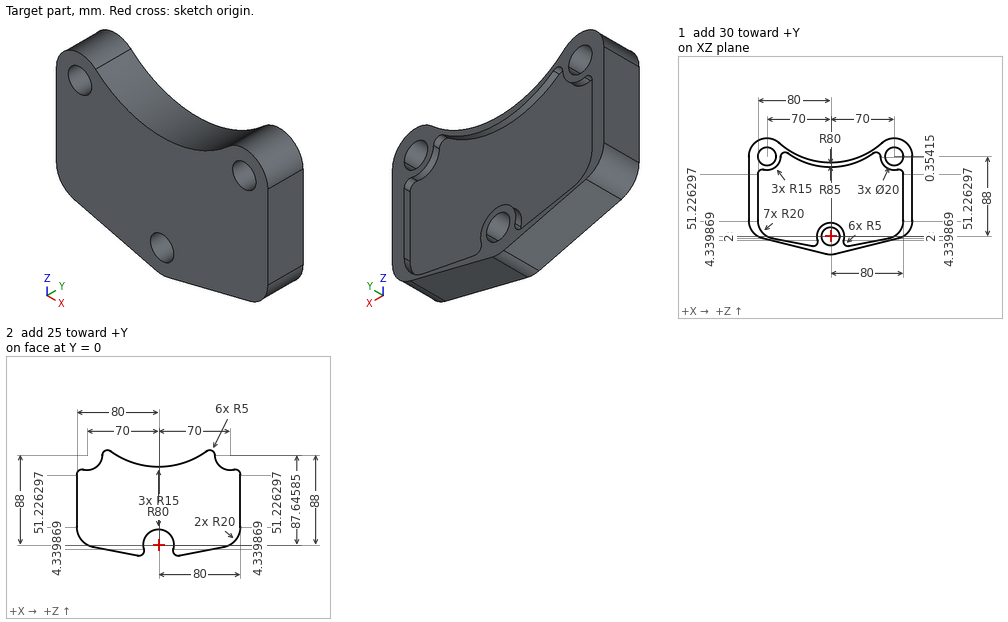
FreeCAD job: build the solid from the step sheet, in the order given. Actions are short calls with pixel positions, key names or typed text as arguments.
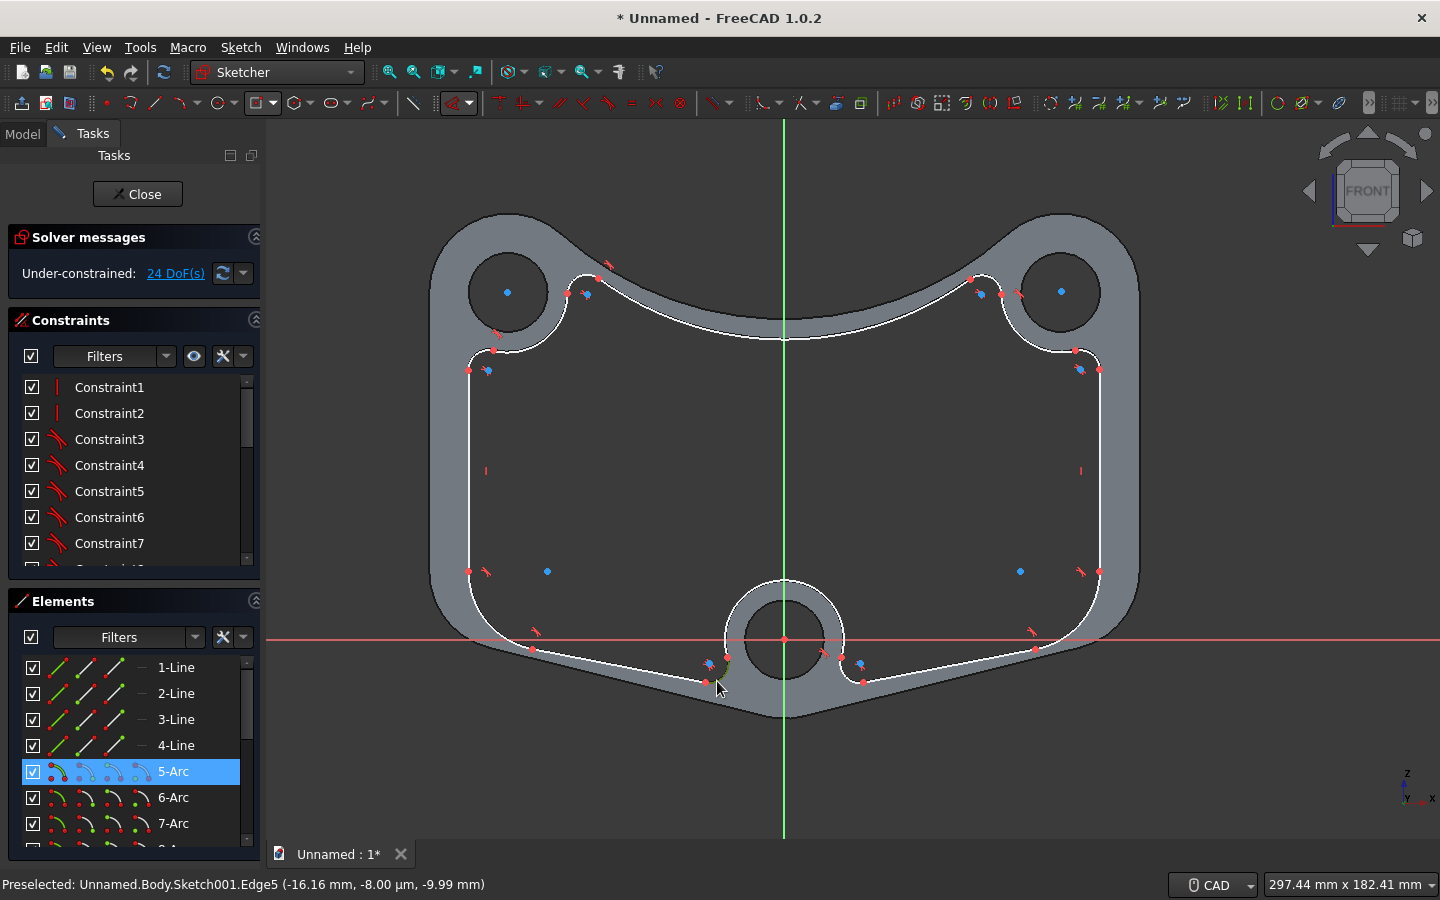
click(841, 669)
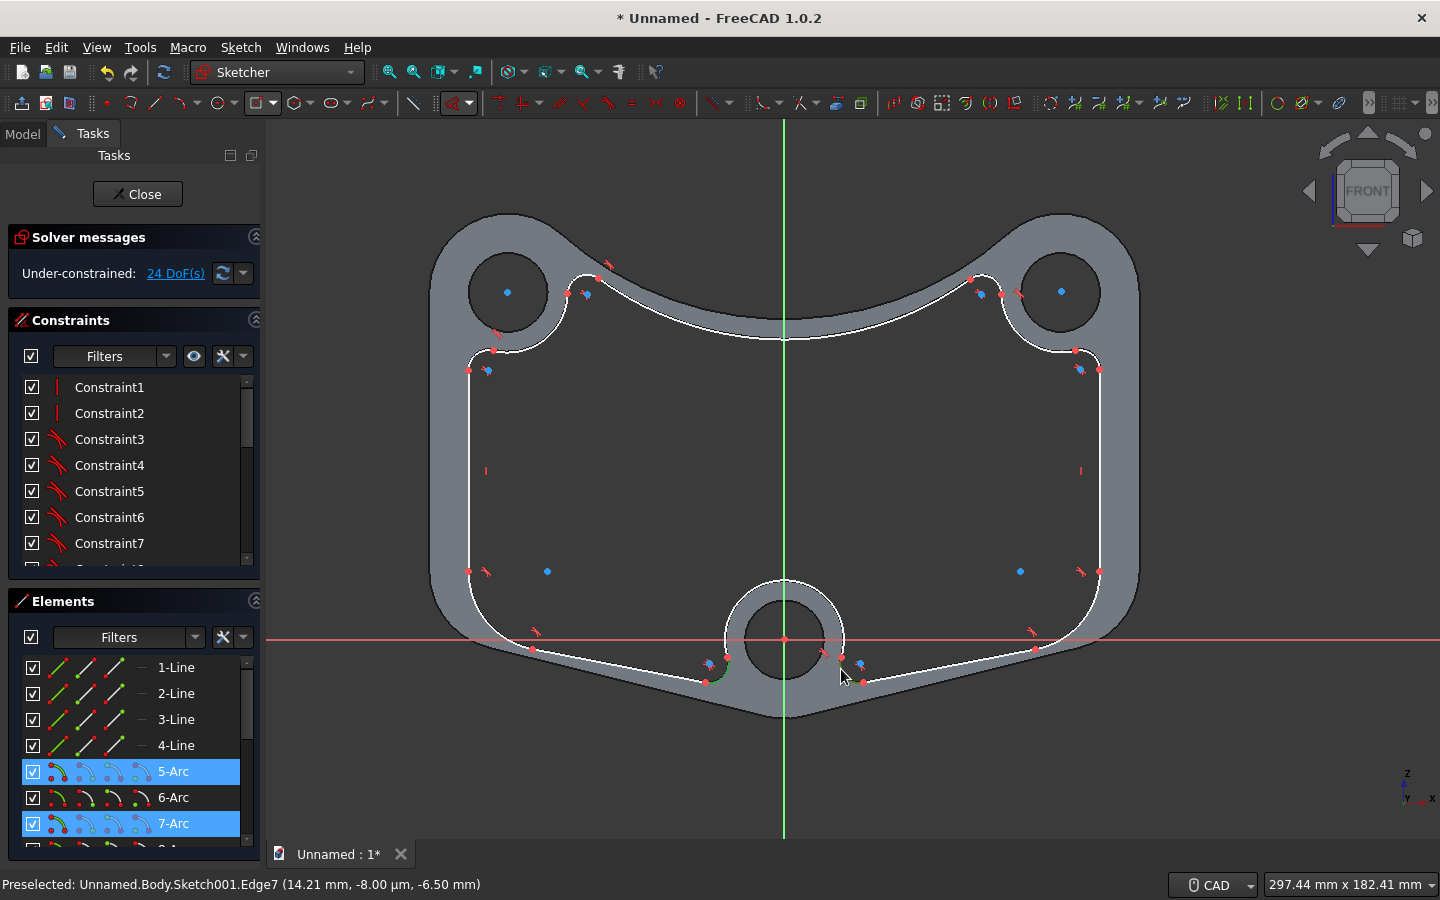
scroll(1097, 360, up, 2)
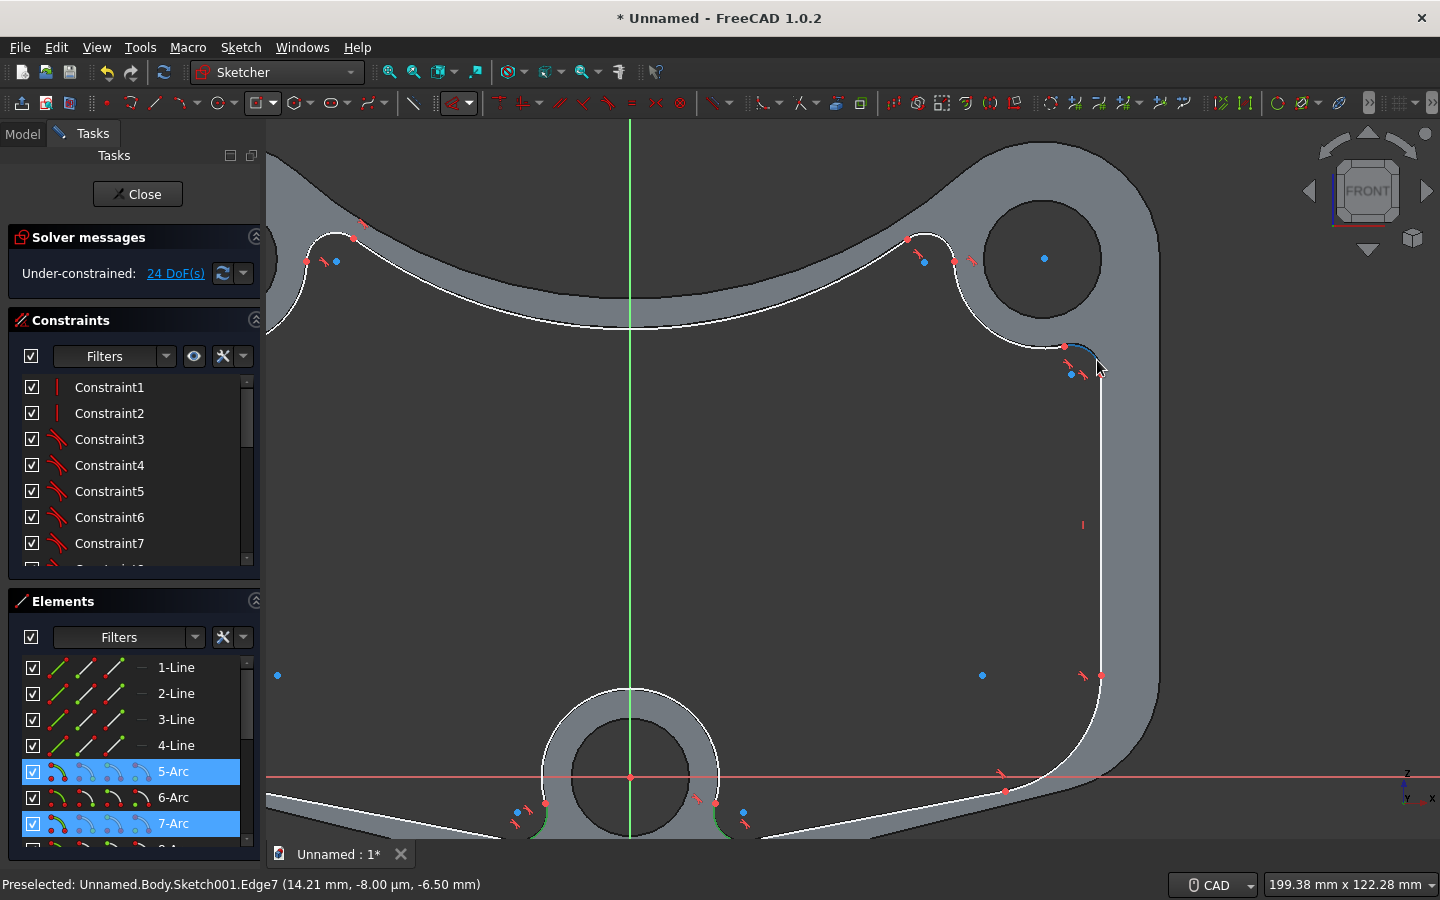
click(1097, 360)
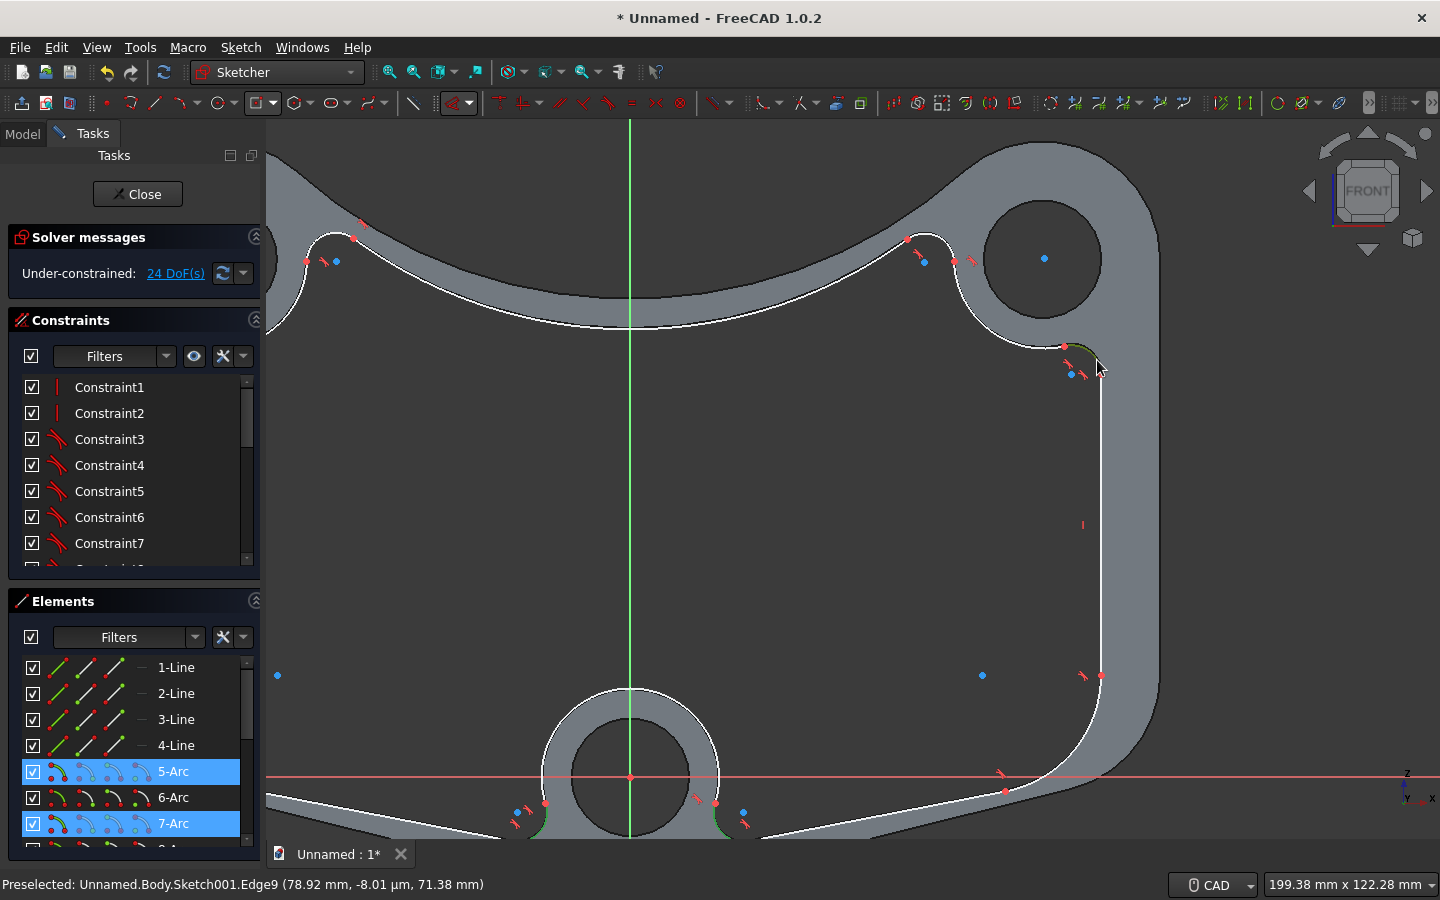
click(947, 244)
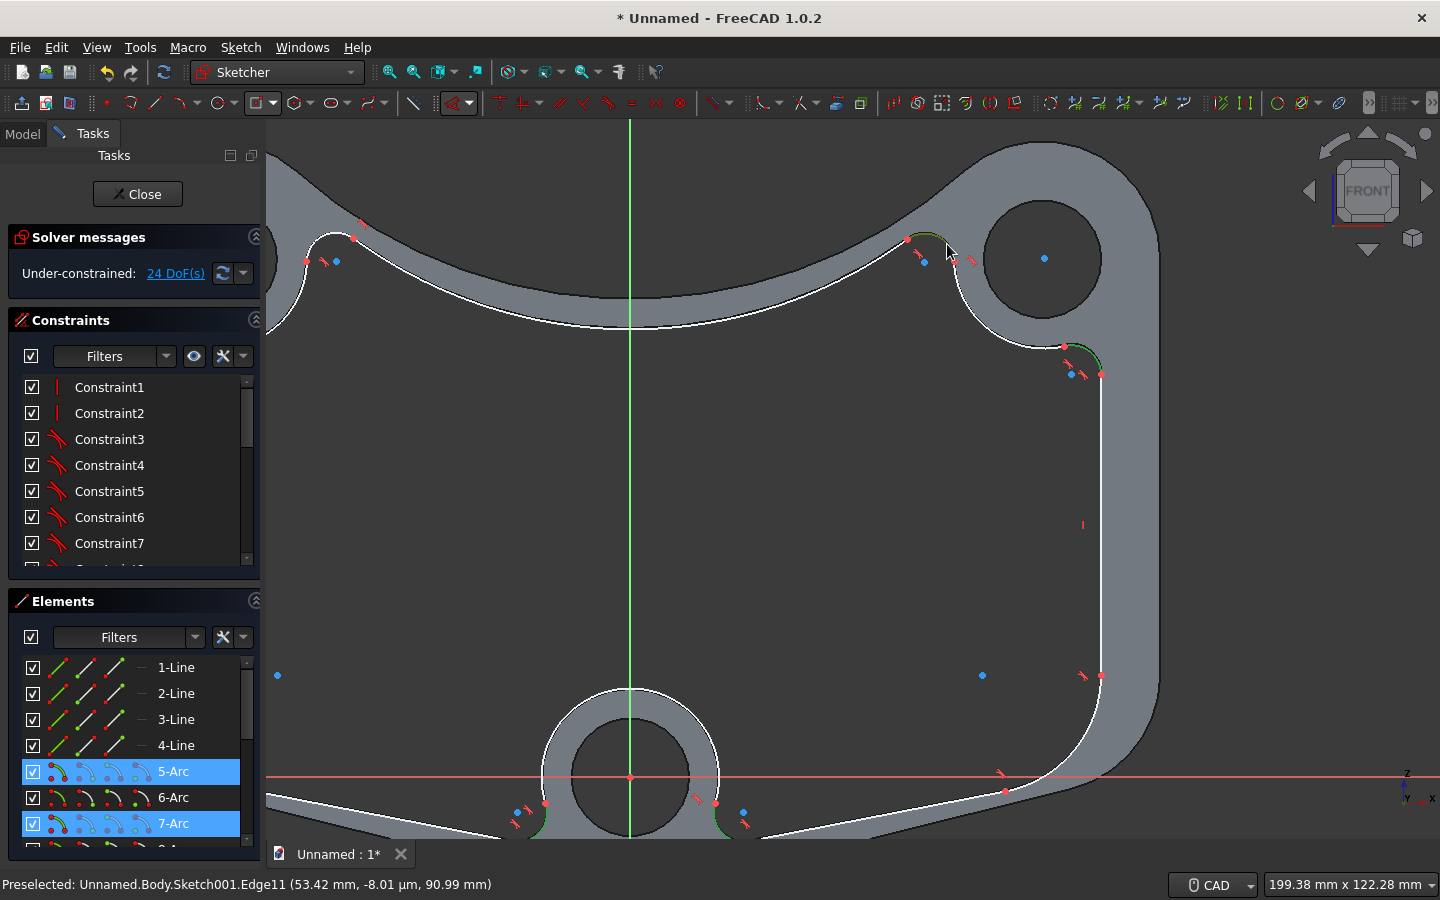
click(335, 233)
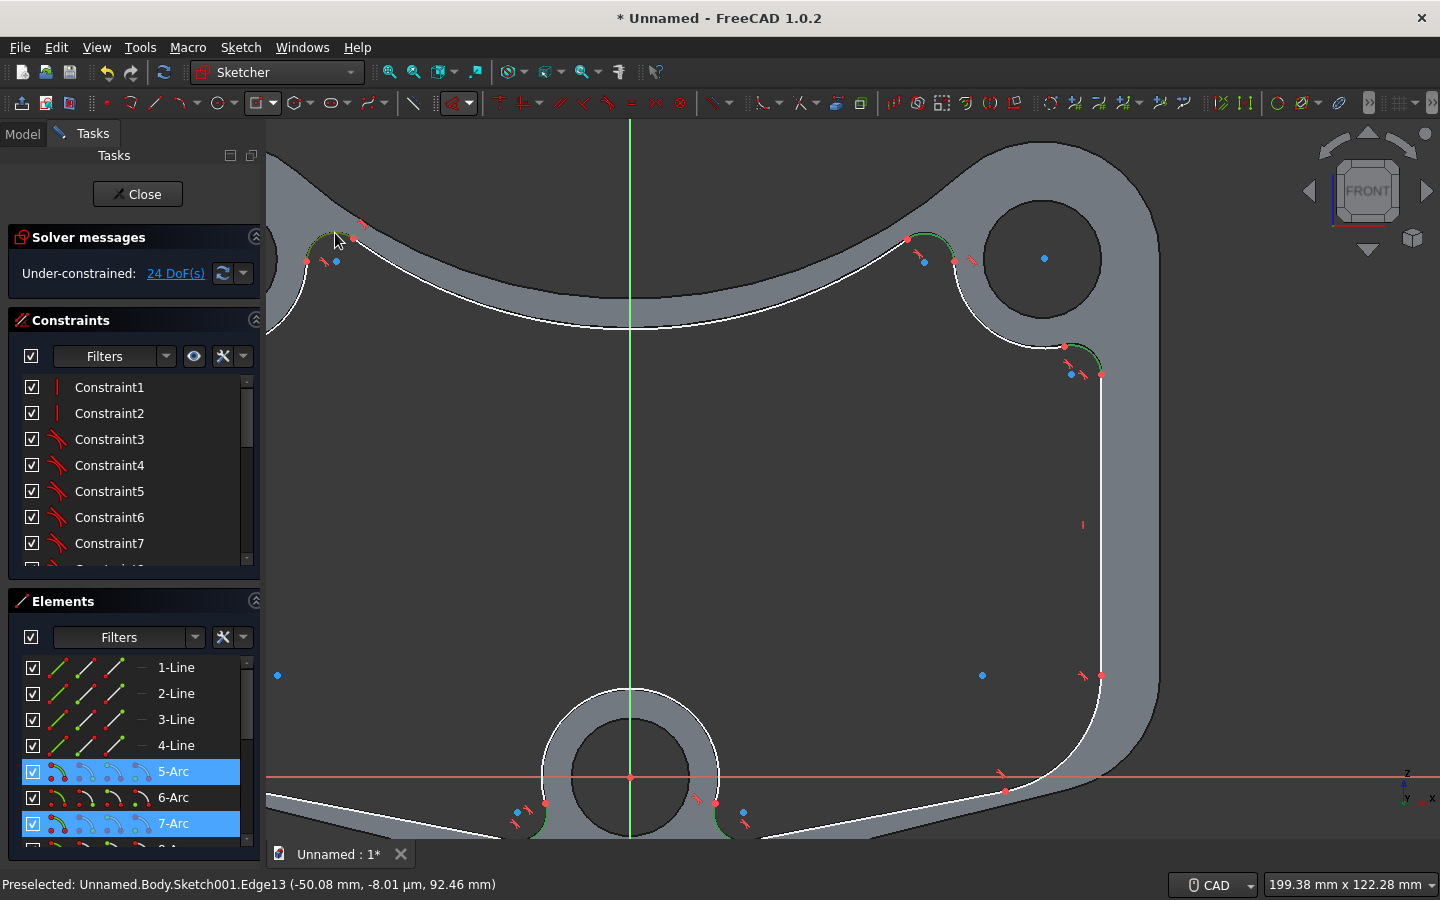
scroll(1098, 359, down, 2)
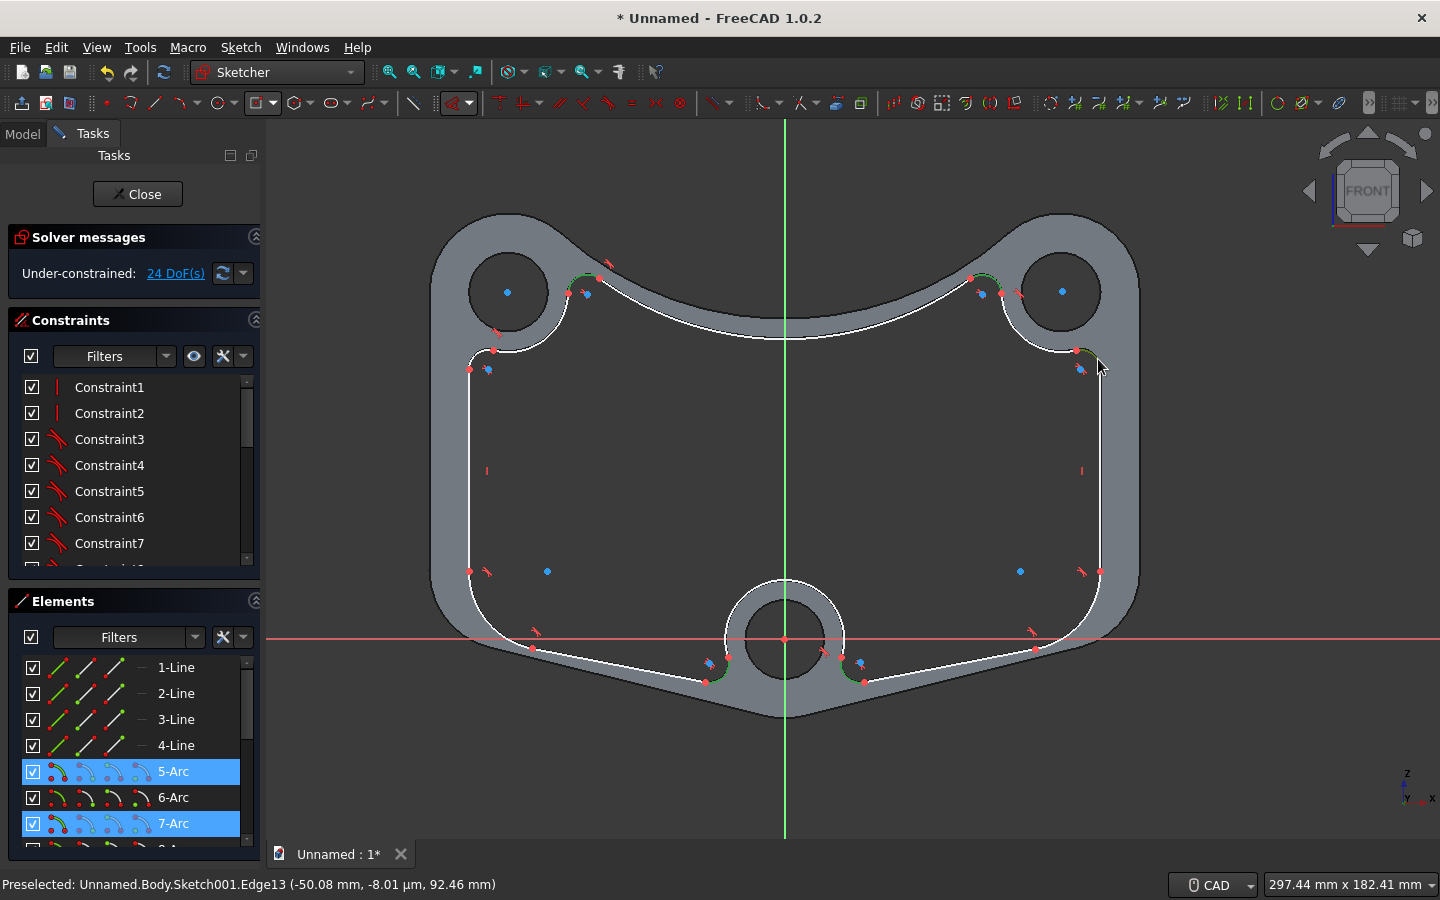
scroll(483, 351, up, 2)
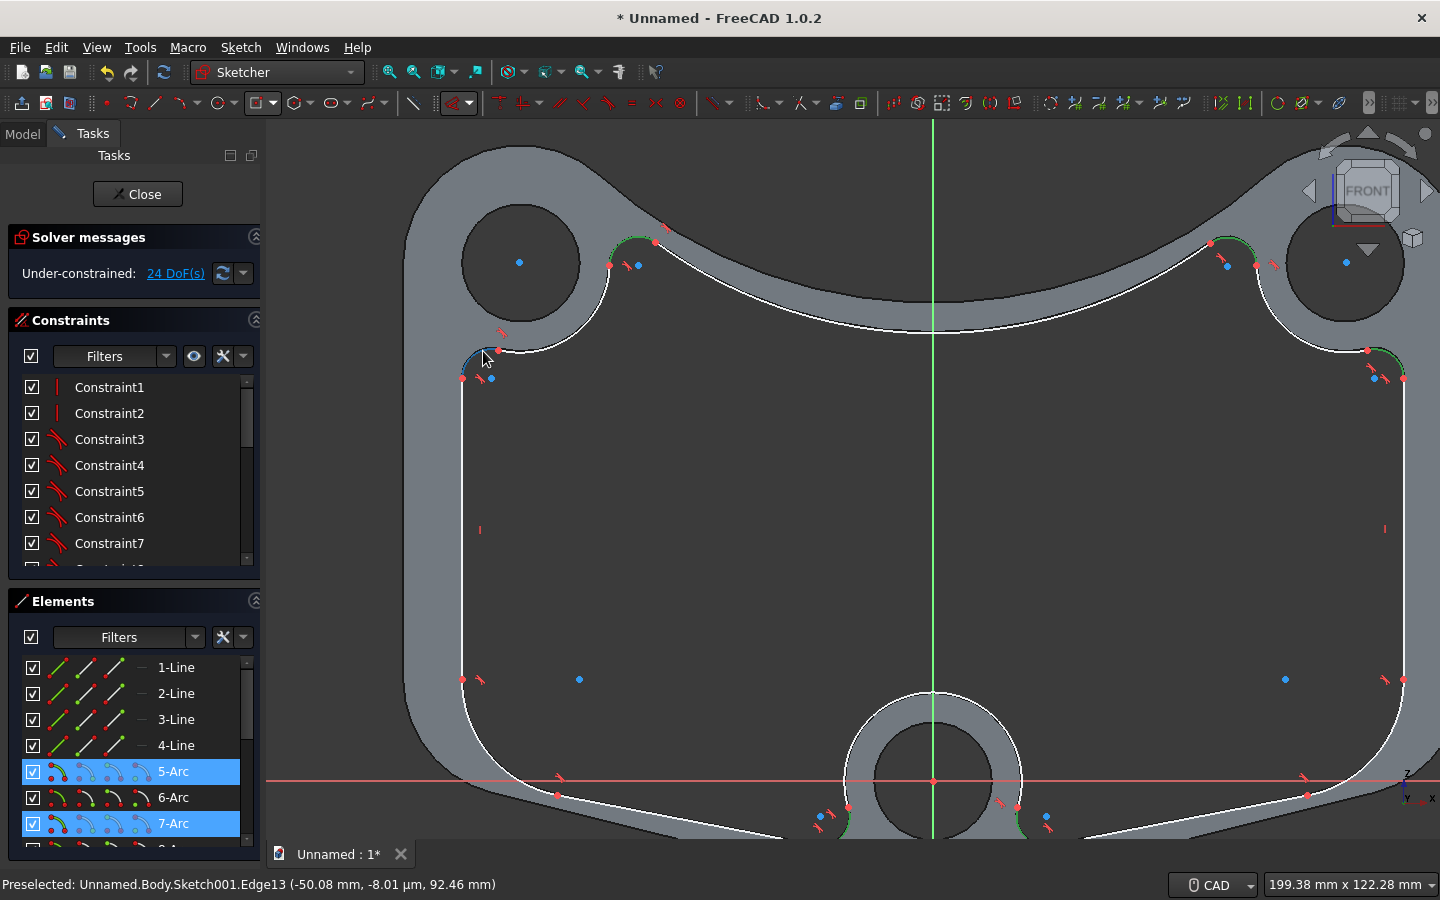
click(483, 351)